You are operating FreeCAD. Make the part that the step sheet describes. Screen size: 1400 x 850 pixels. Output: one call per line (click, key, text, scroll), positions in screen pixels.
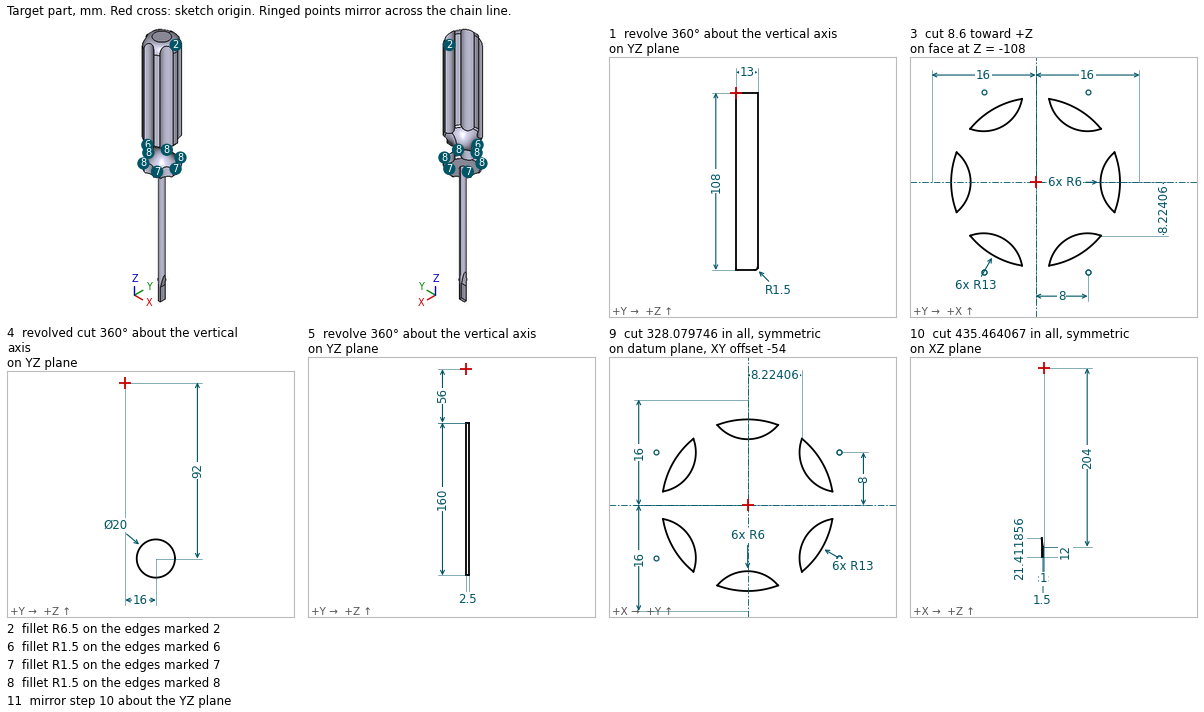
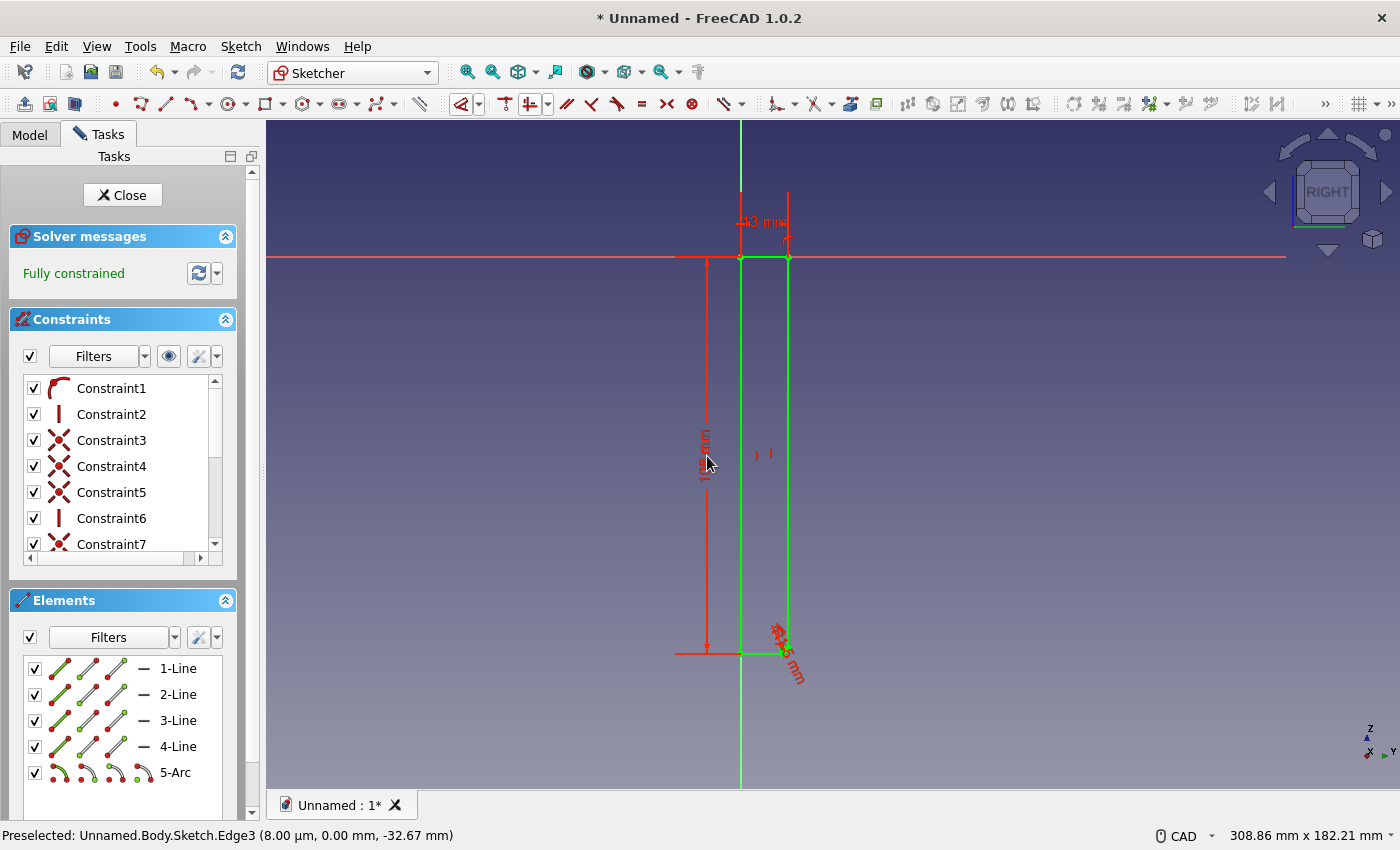
click(123, 195)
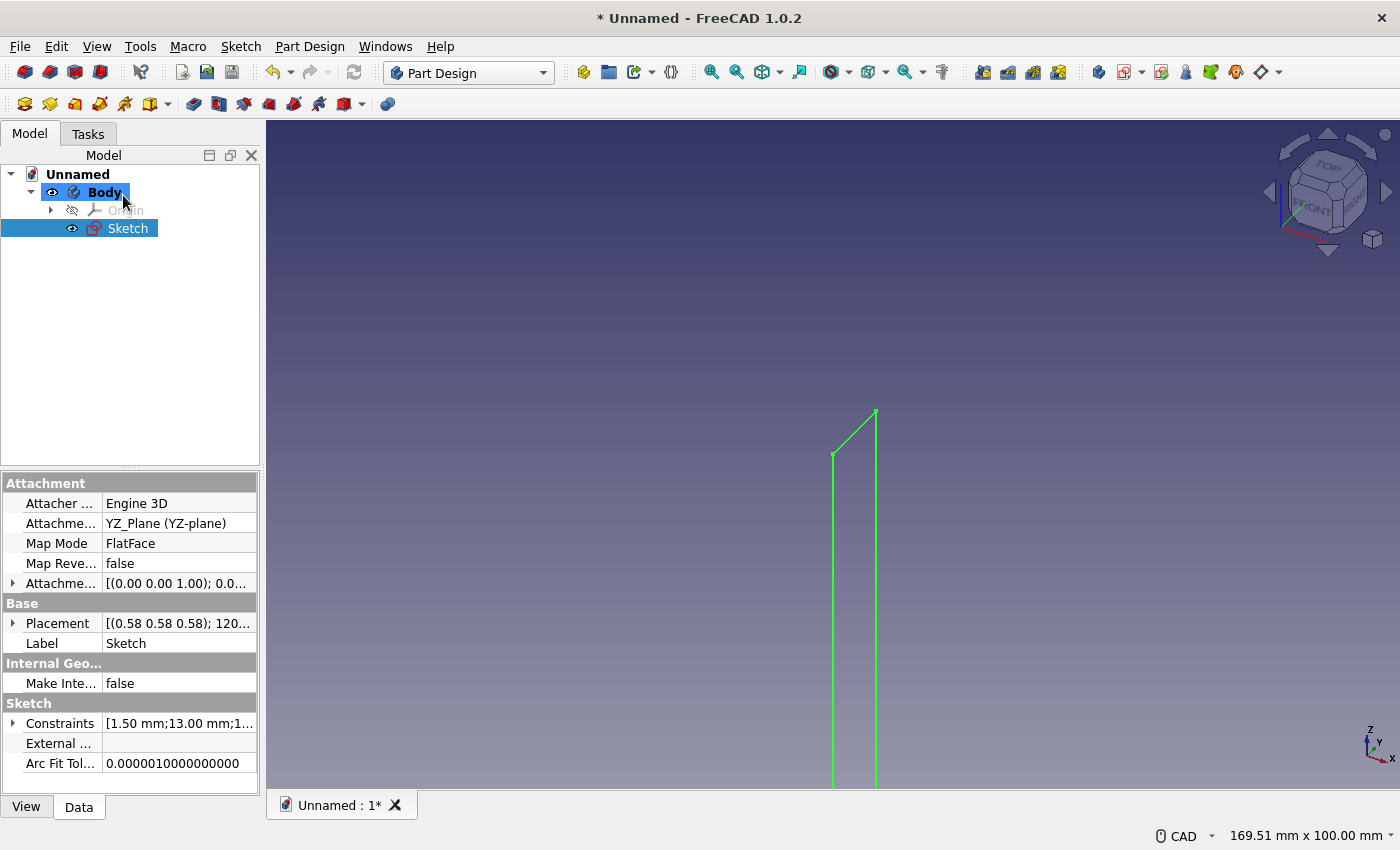
click(50, 104)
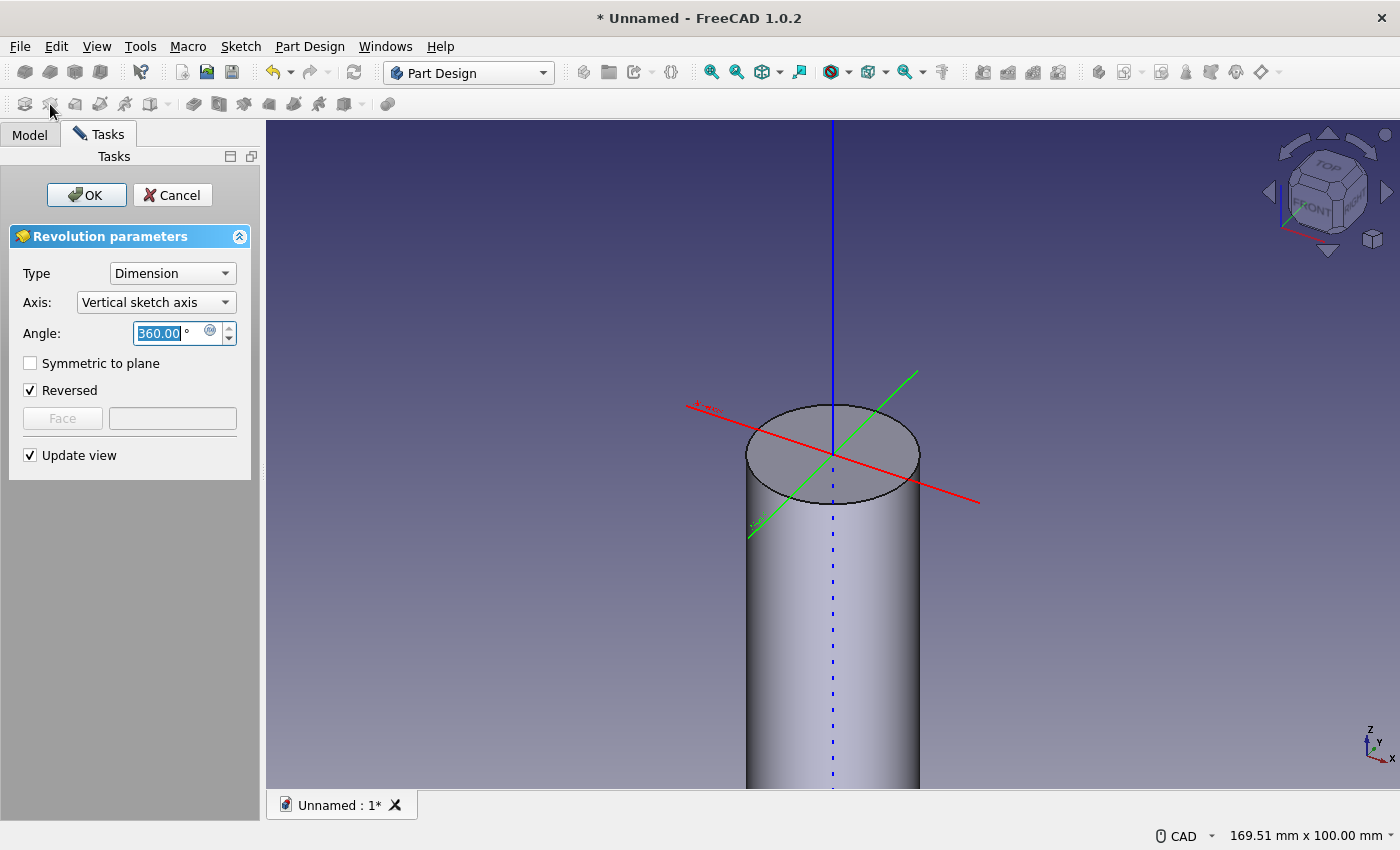
click(87, 195)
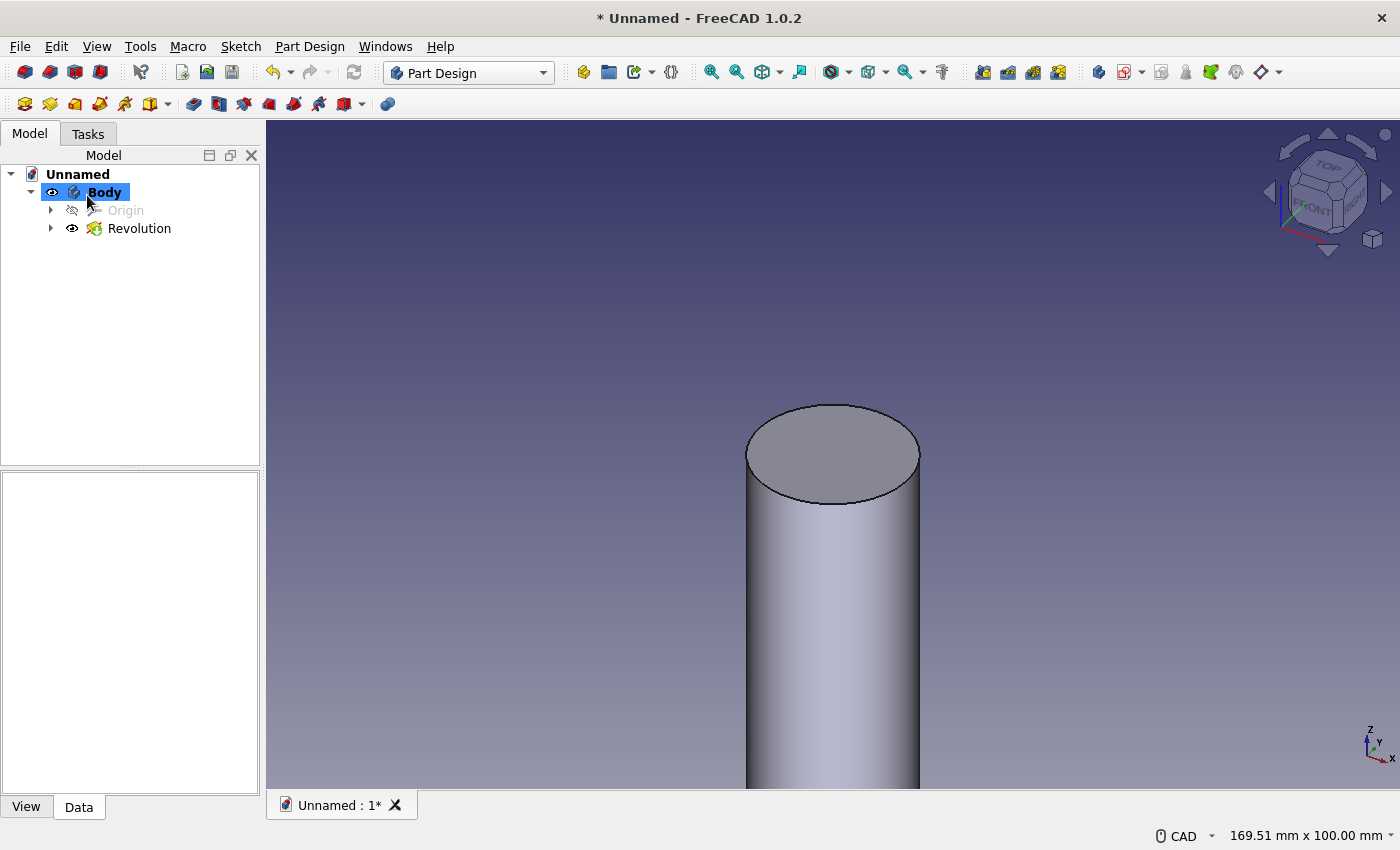
key(v)
key(f)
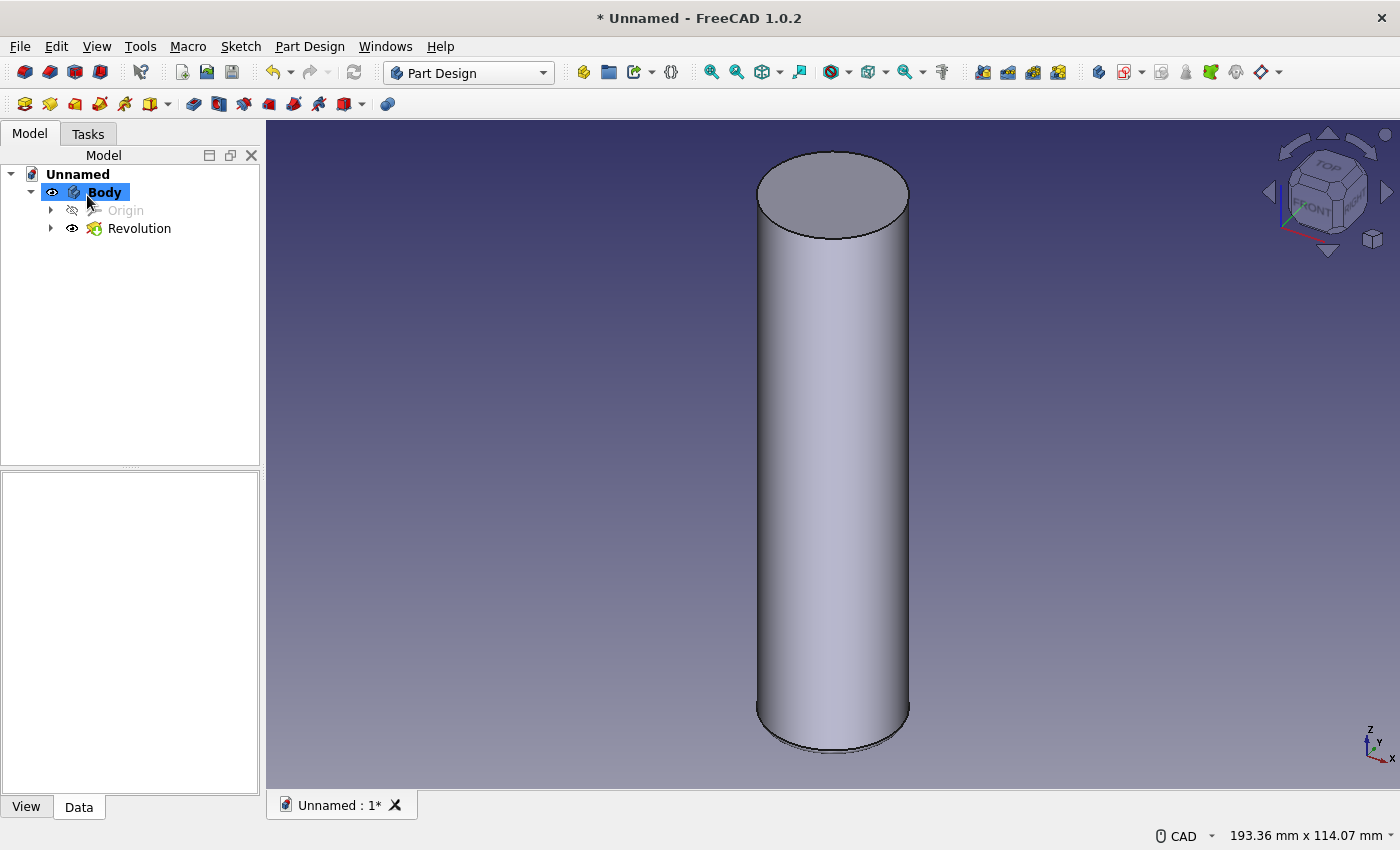
click(795, 232)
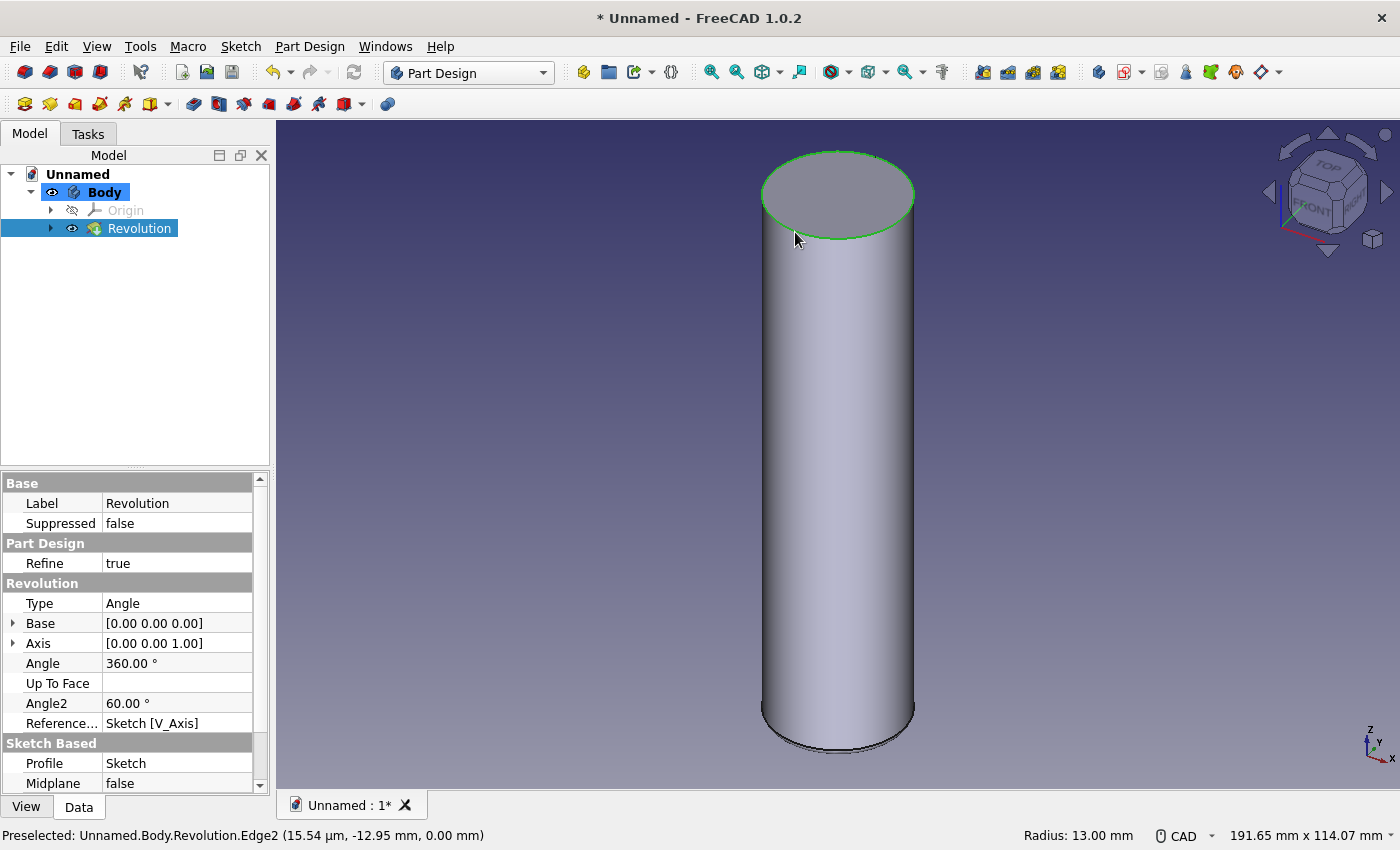
click(25, 72)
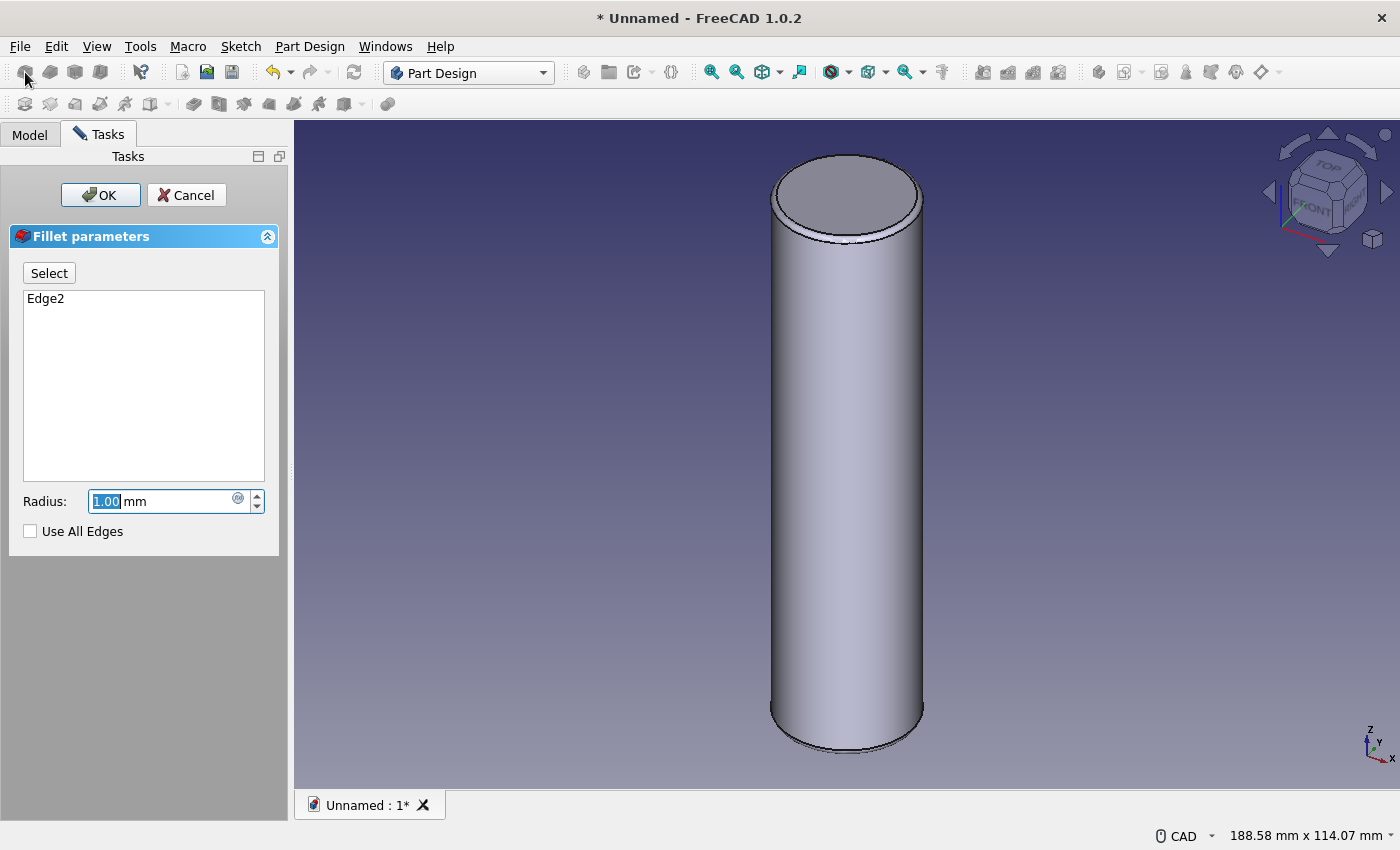
text(6.5)
key(Tab)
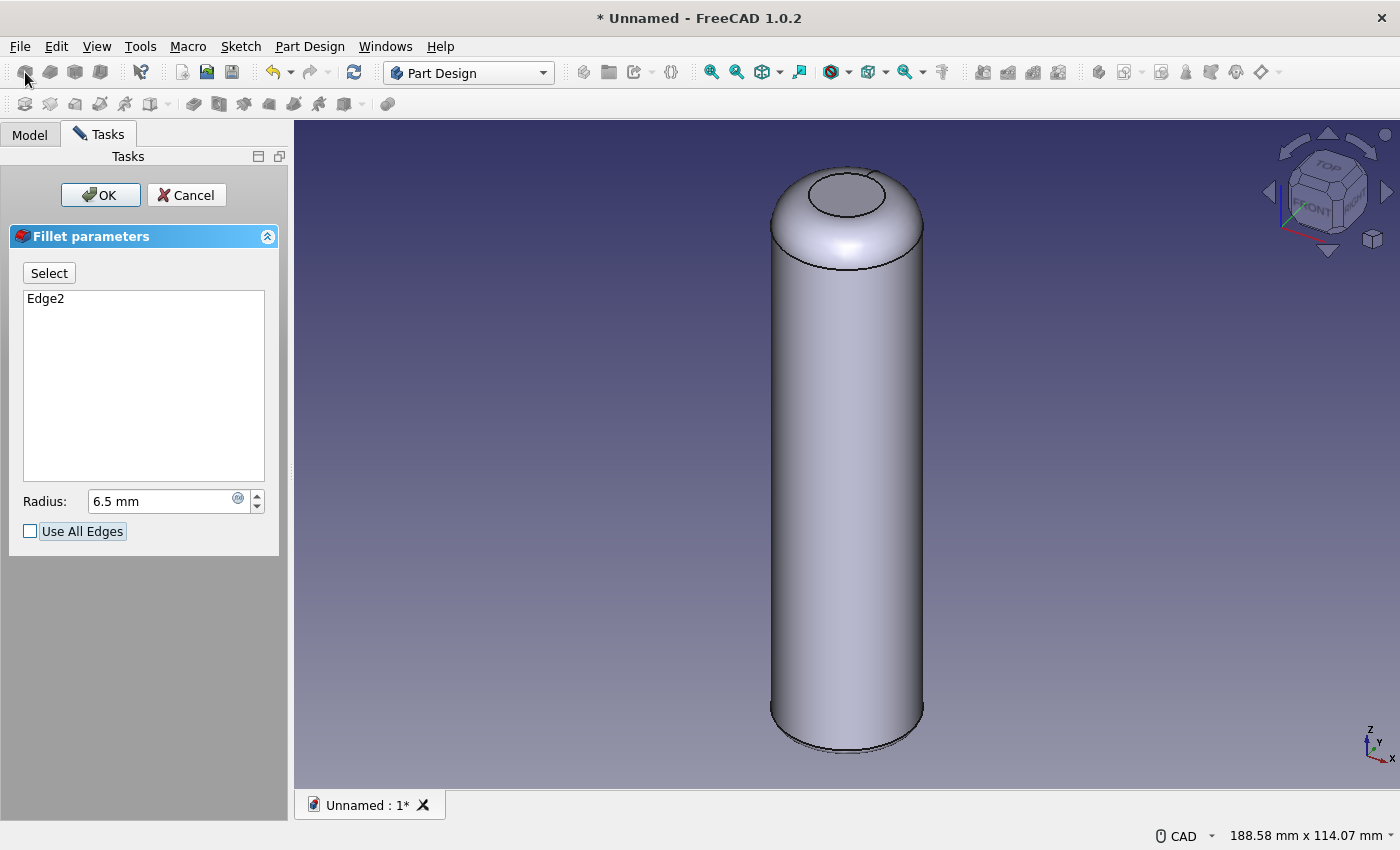
click(101, 195)